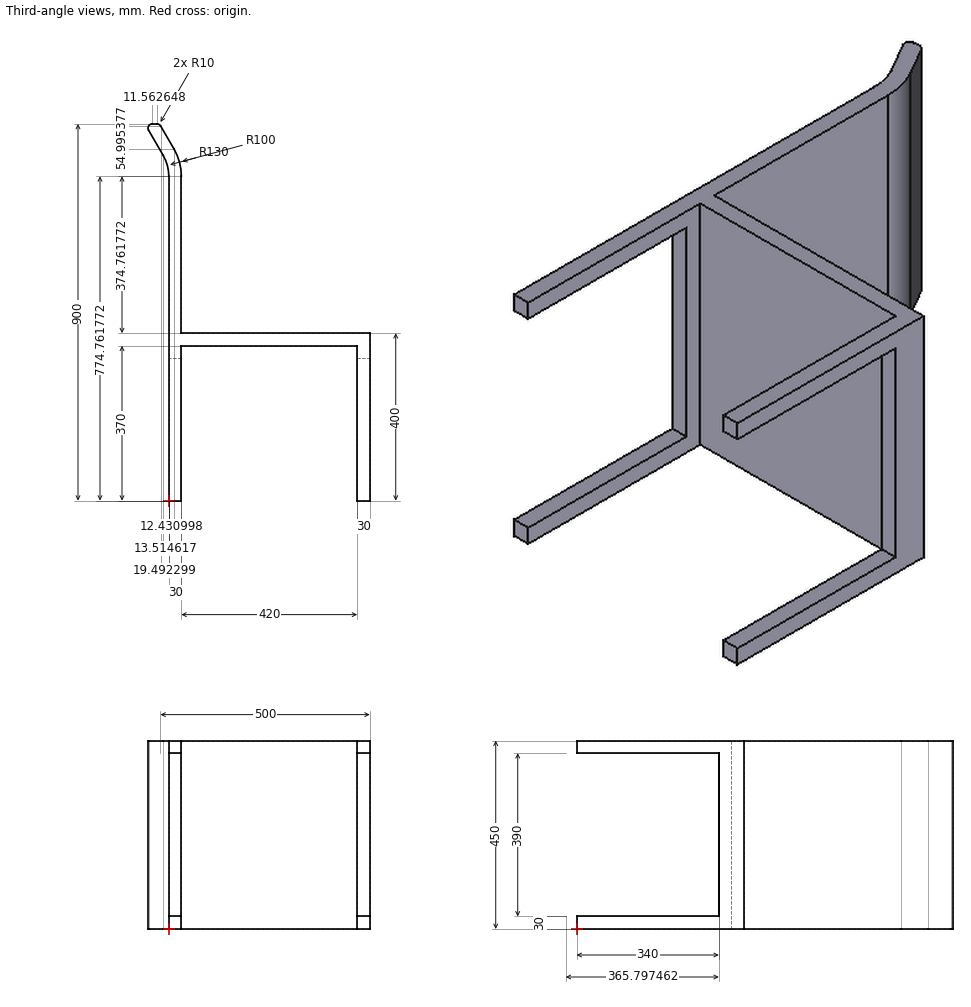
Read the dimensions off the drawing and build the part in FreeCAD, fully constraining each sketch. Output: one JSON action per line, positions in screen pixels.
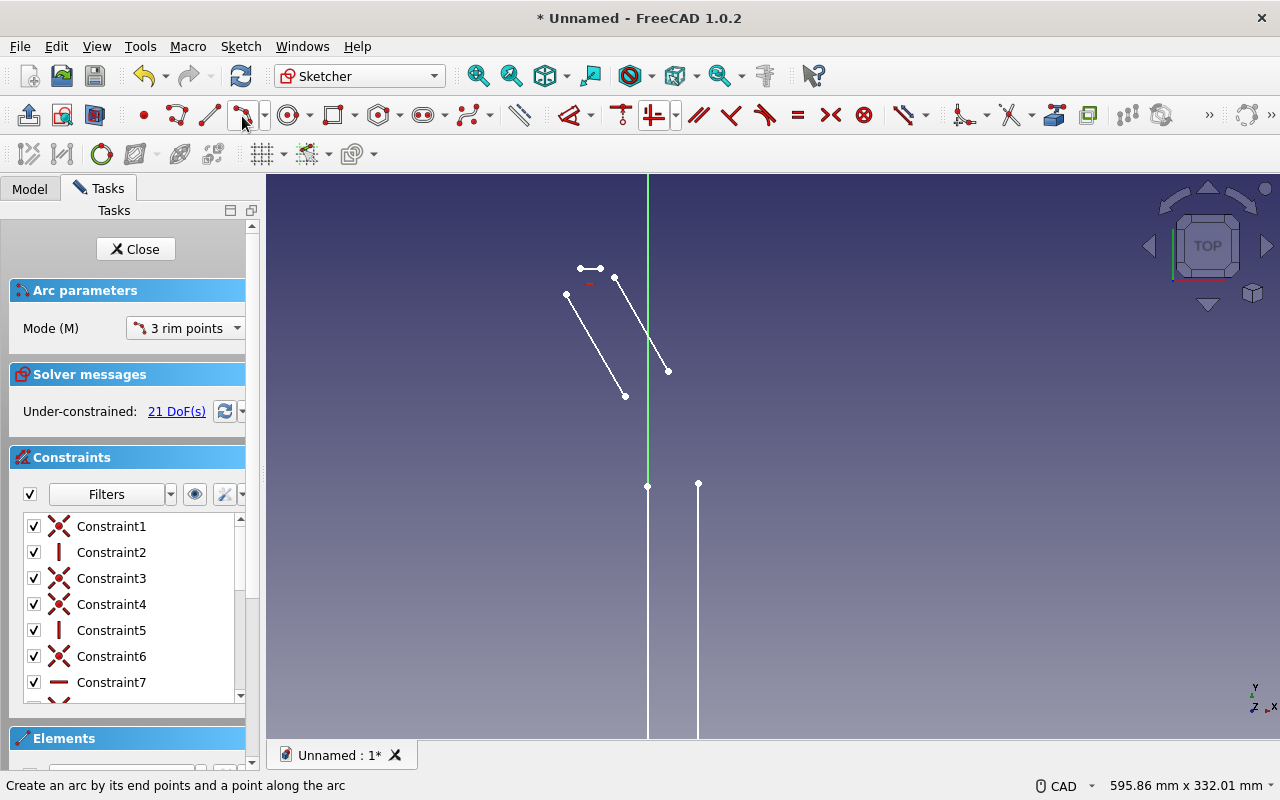
{"action": "scroll", "coordinate": [603, 268], "scroll_direction": "down", "scroll_amount": 7}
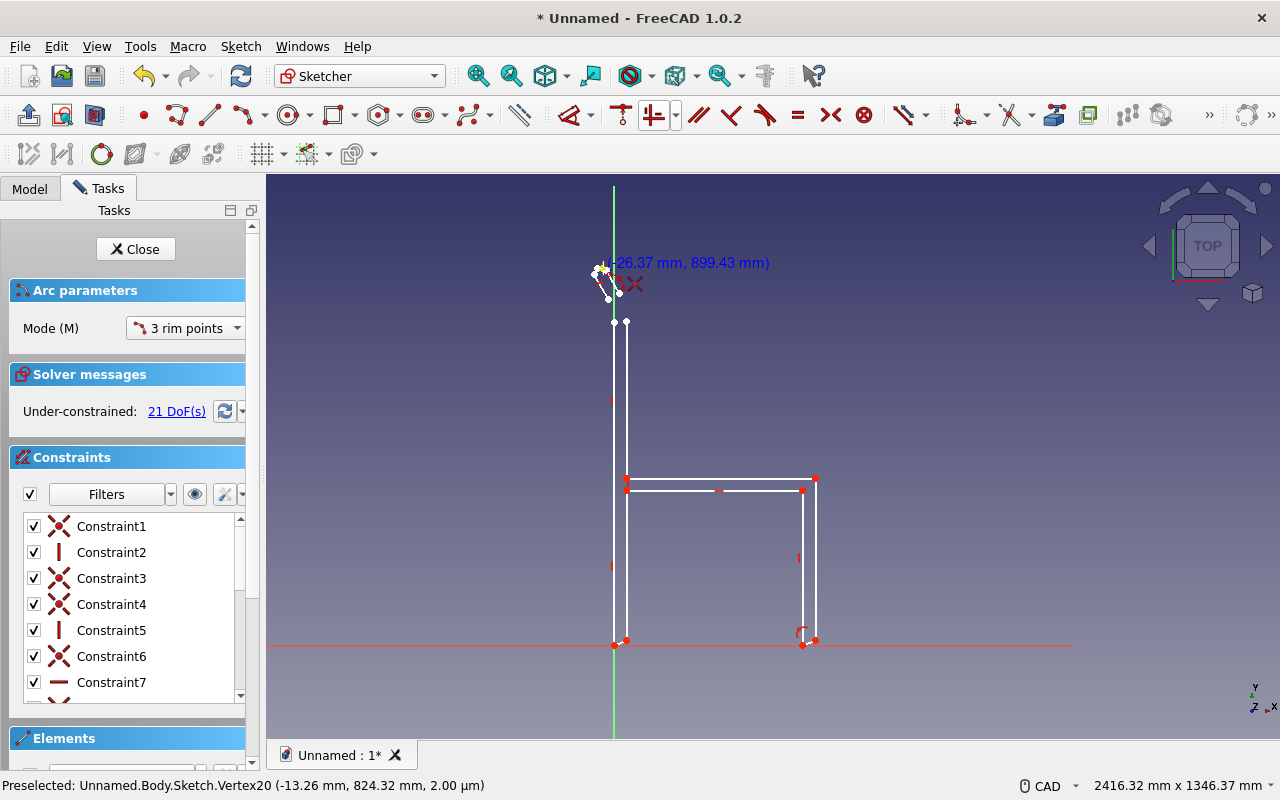
{"action": "scroll", "coordinate": [627, 321], "scroll_direction": "up", "scroll_amount": 2}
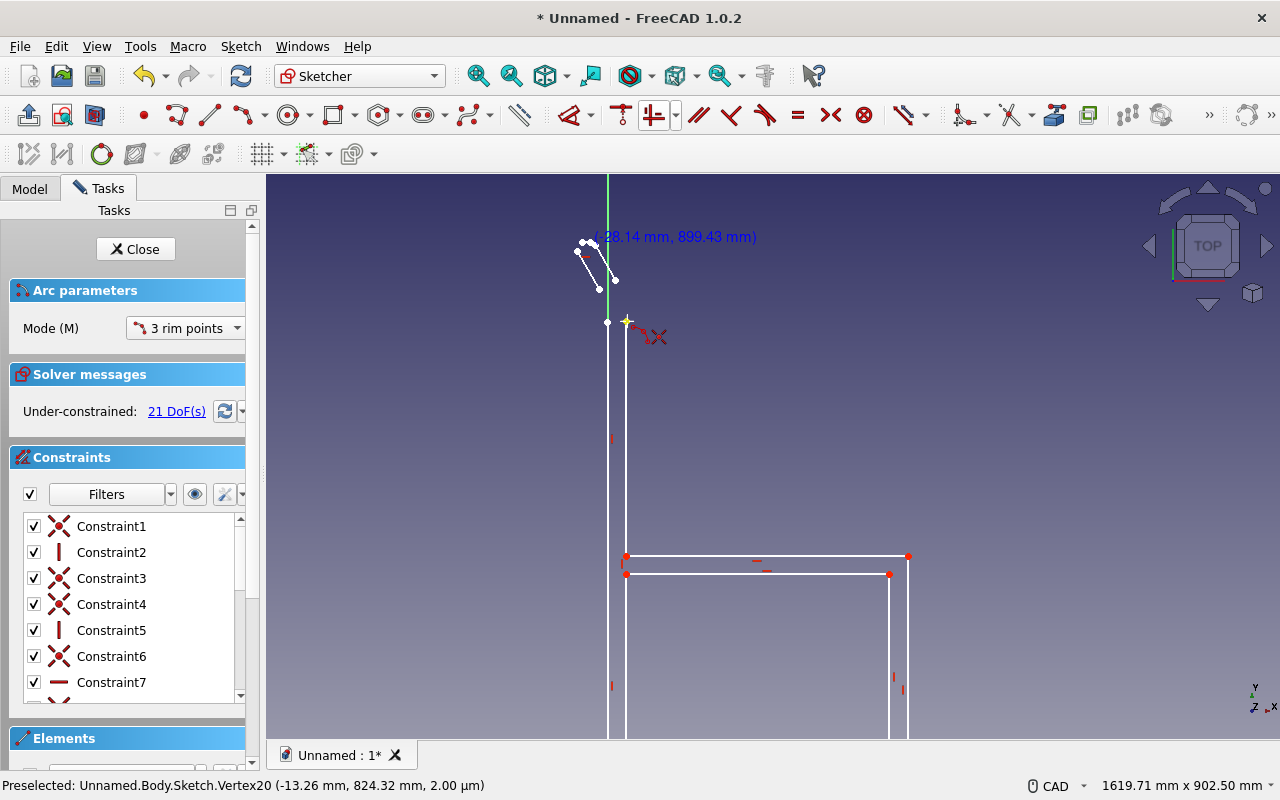
{"action": "left_click", "coordinate": [626, 321]}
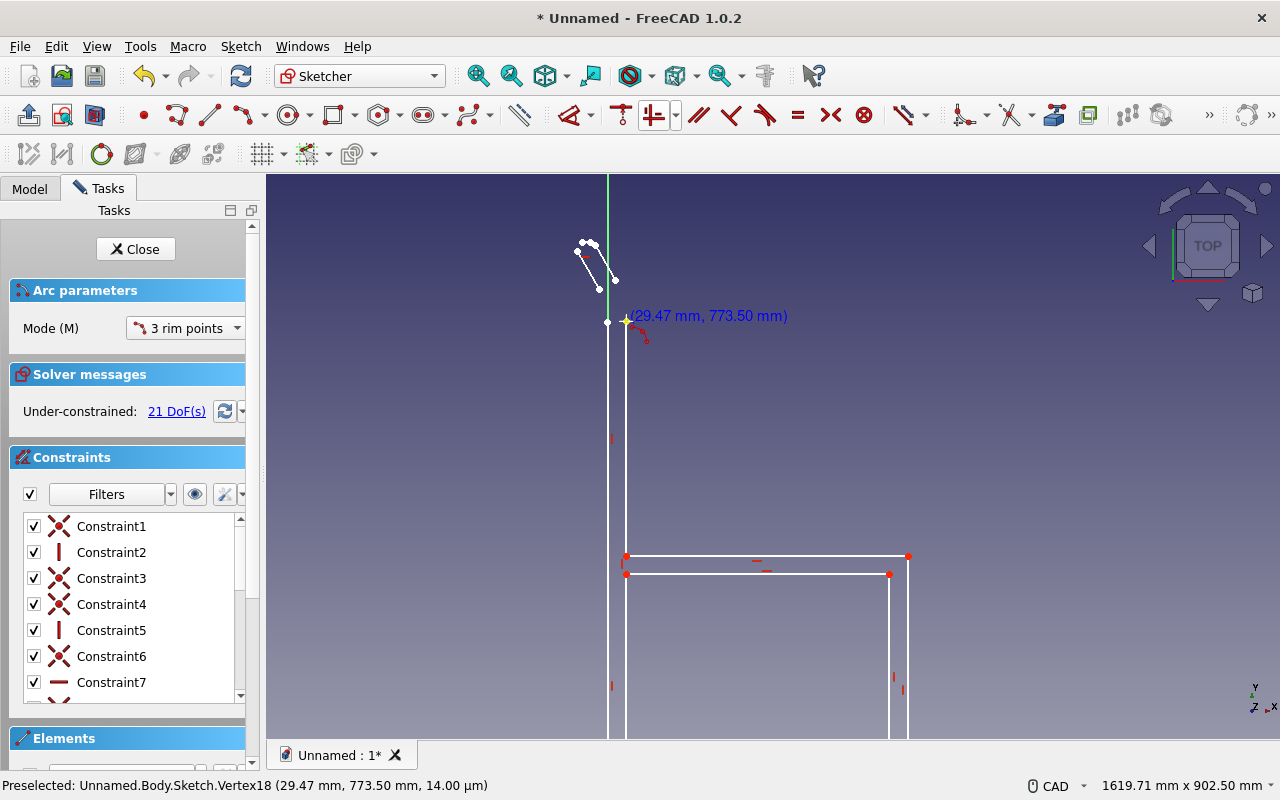
{"action": "scroll", "coordinate": [616, 280], "scroll_direction": "up", "scroll_amount": 4}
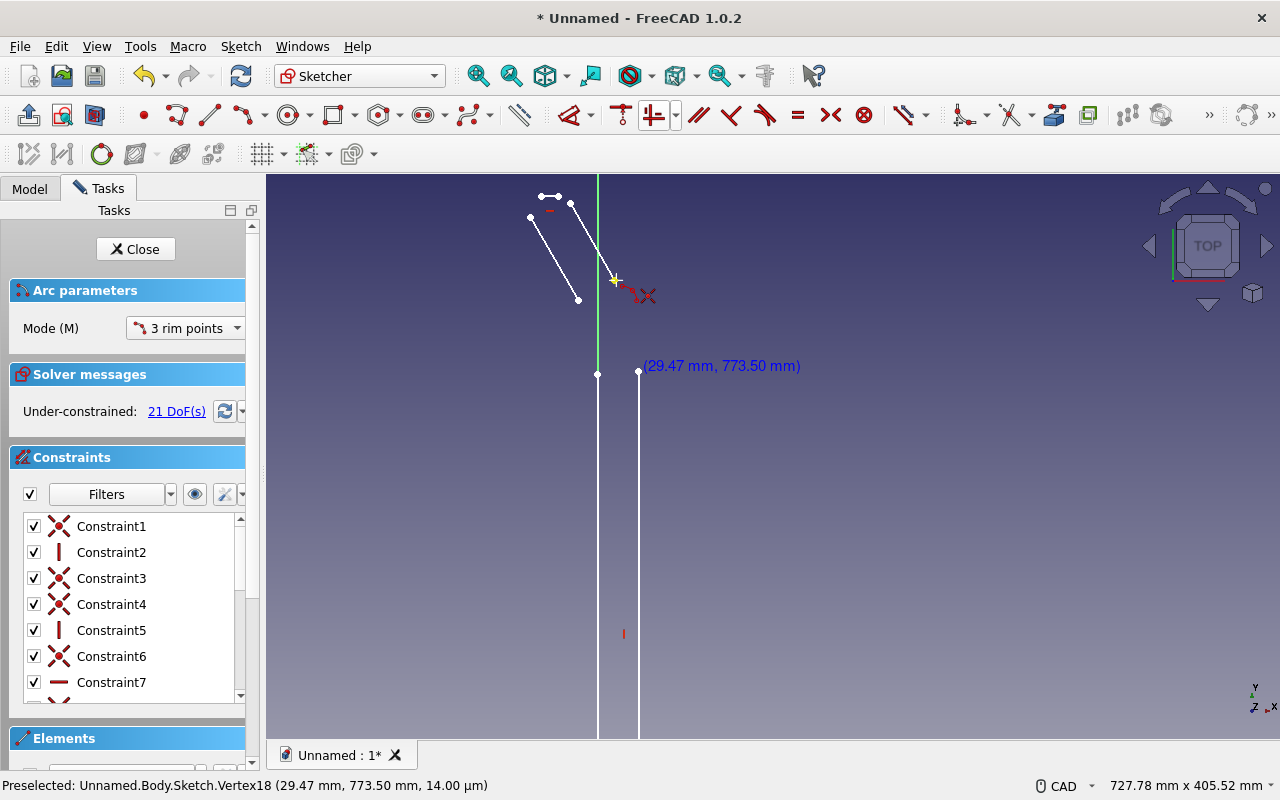
{"action": "left_click", "coordinate": [615, 280]}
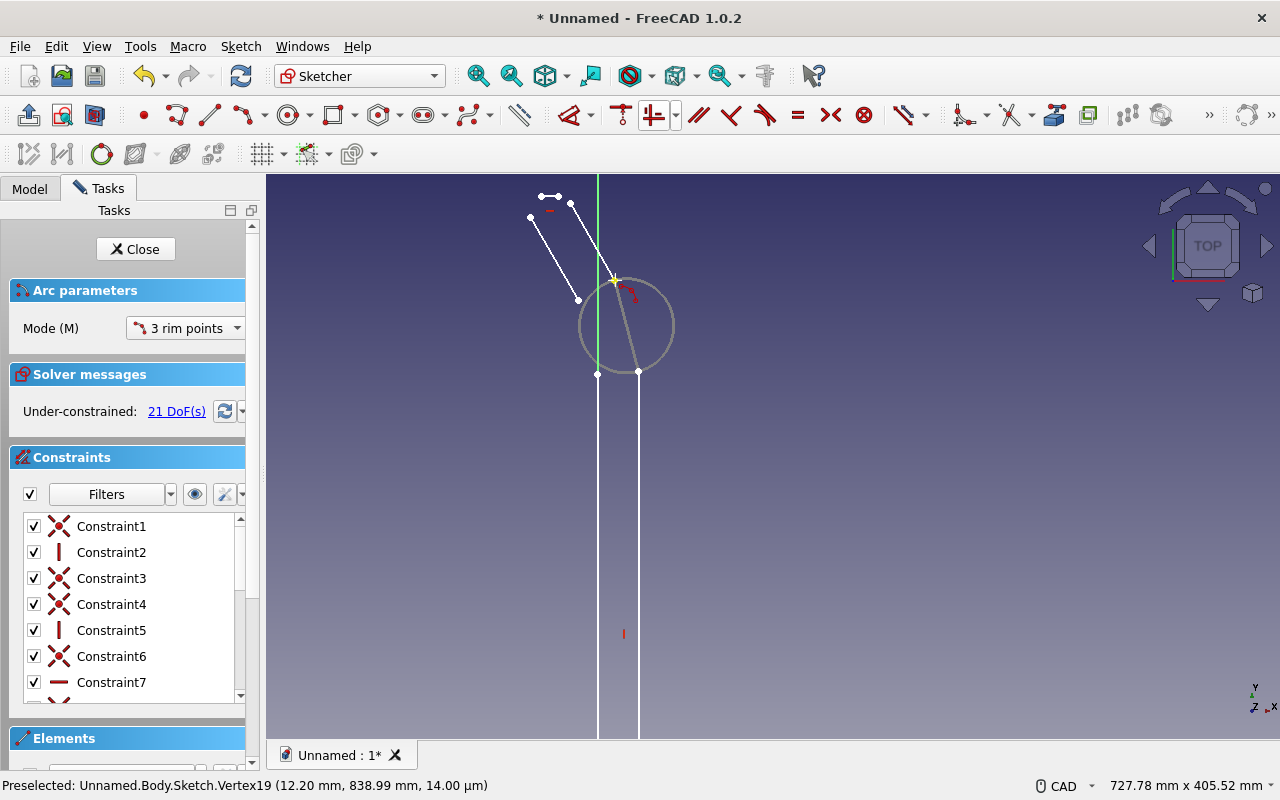
{"action": "scroll", "coordinate": [633, 323], "scroll_direction": "up", "scroll_amount": 5}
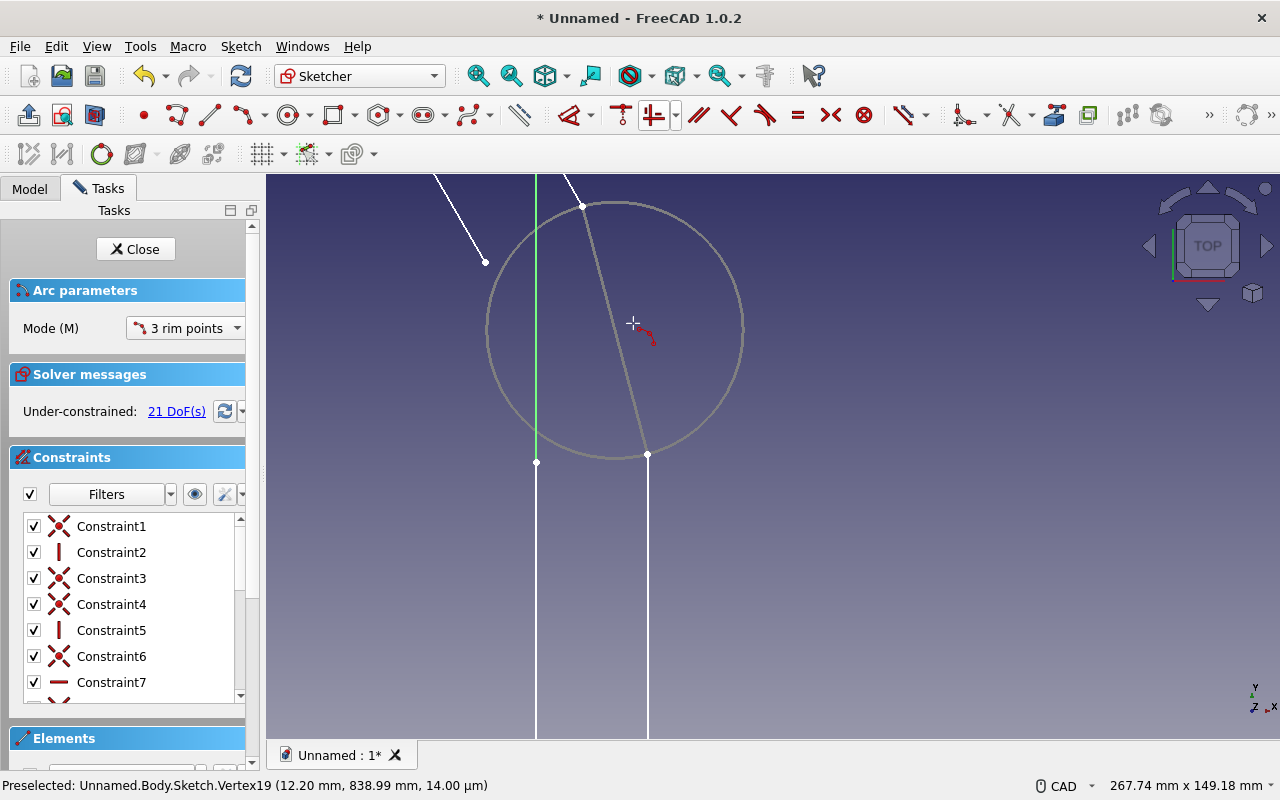
{"action": "left_click", "coordinate": [633, 321]}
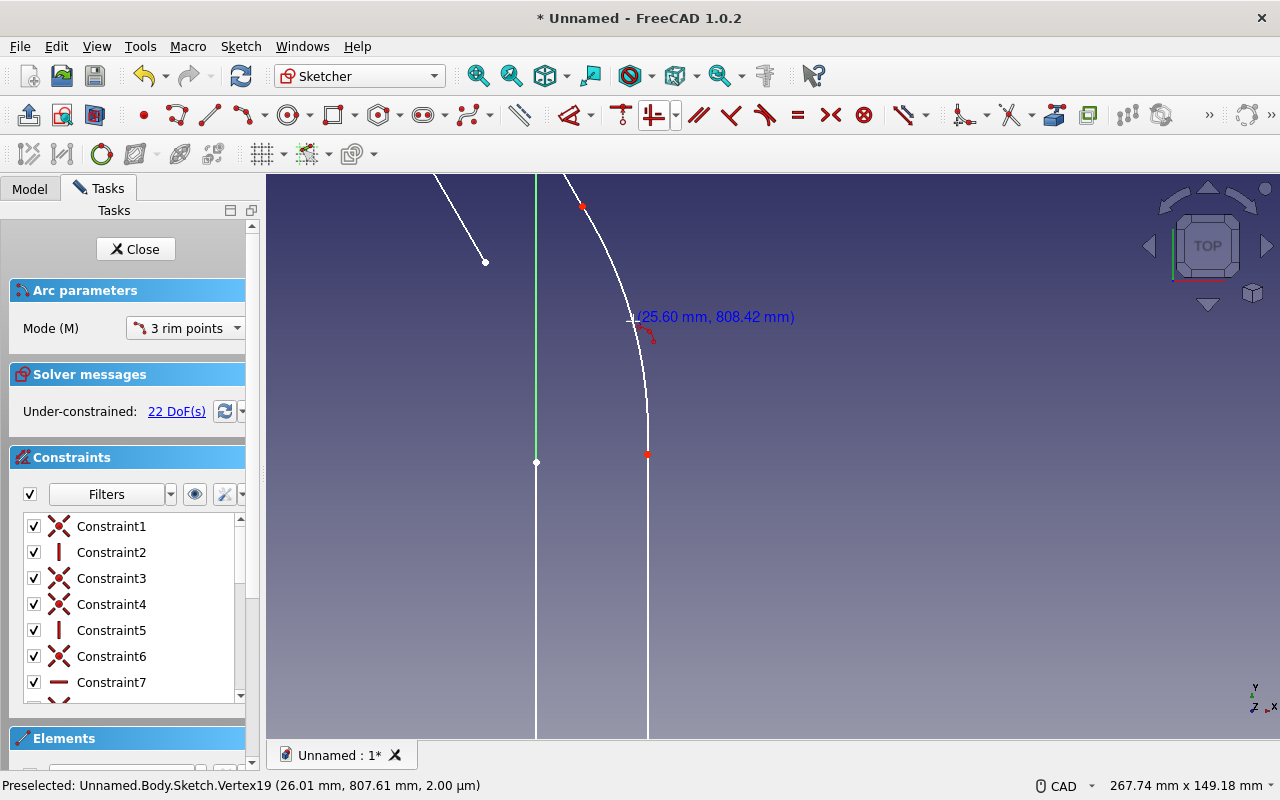
{"action": "scroll", "coordinate": [624, 304], "scroll_direction": "down", "scroll_amount": 11}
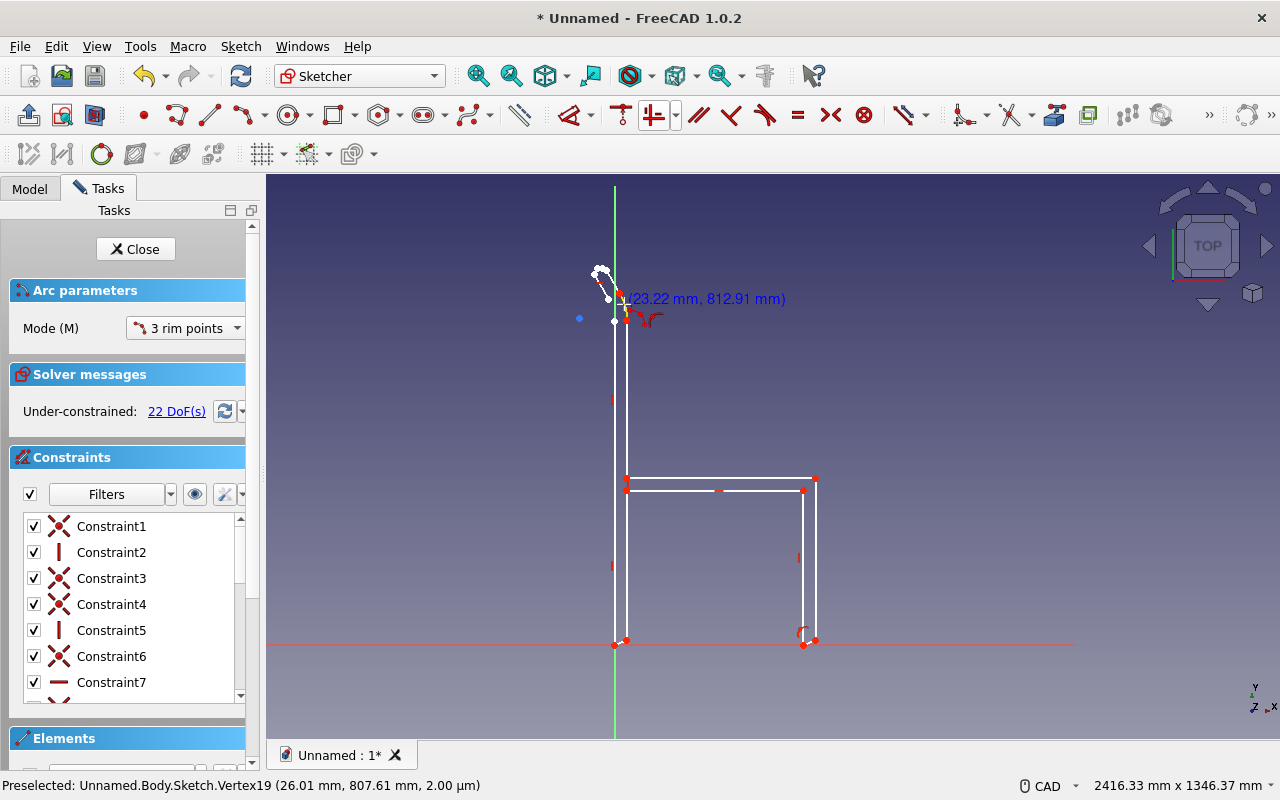
{"action": "scroll", "coordinate": [606, 270], "scroll_direction": "up", "scroll_amount": 7}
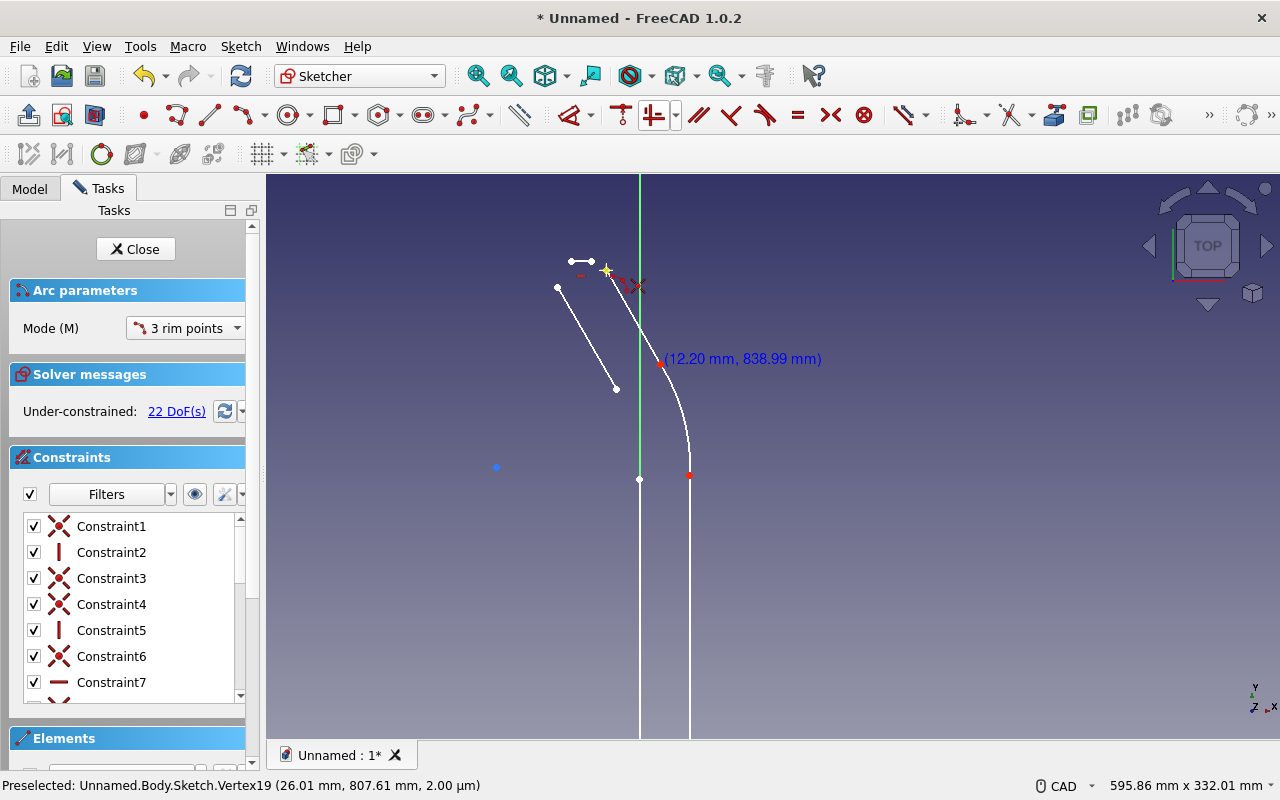
{"action": "left_click", "coordinate": [607, 270]}